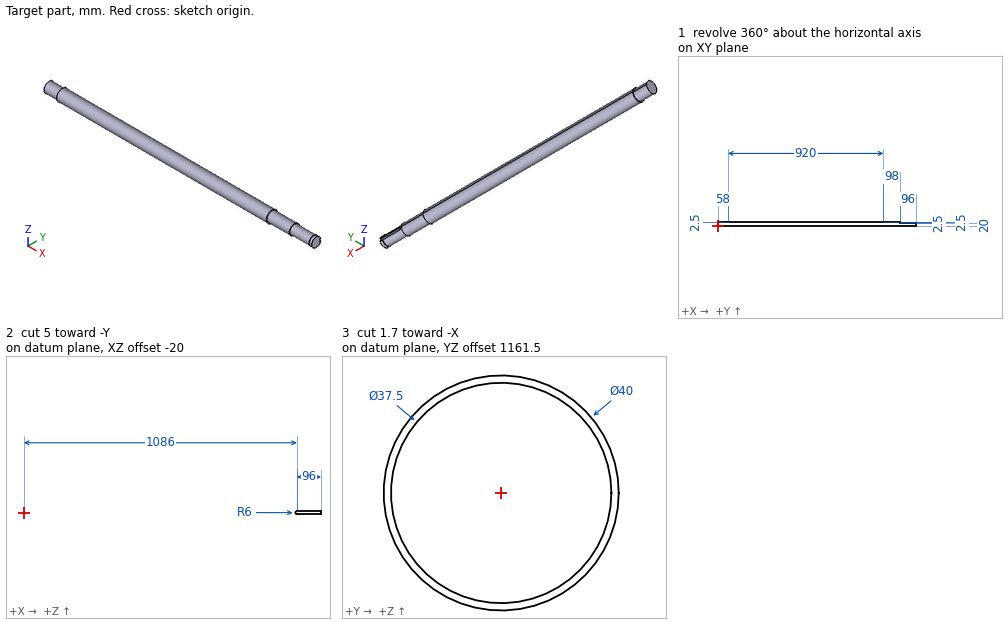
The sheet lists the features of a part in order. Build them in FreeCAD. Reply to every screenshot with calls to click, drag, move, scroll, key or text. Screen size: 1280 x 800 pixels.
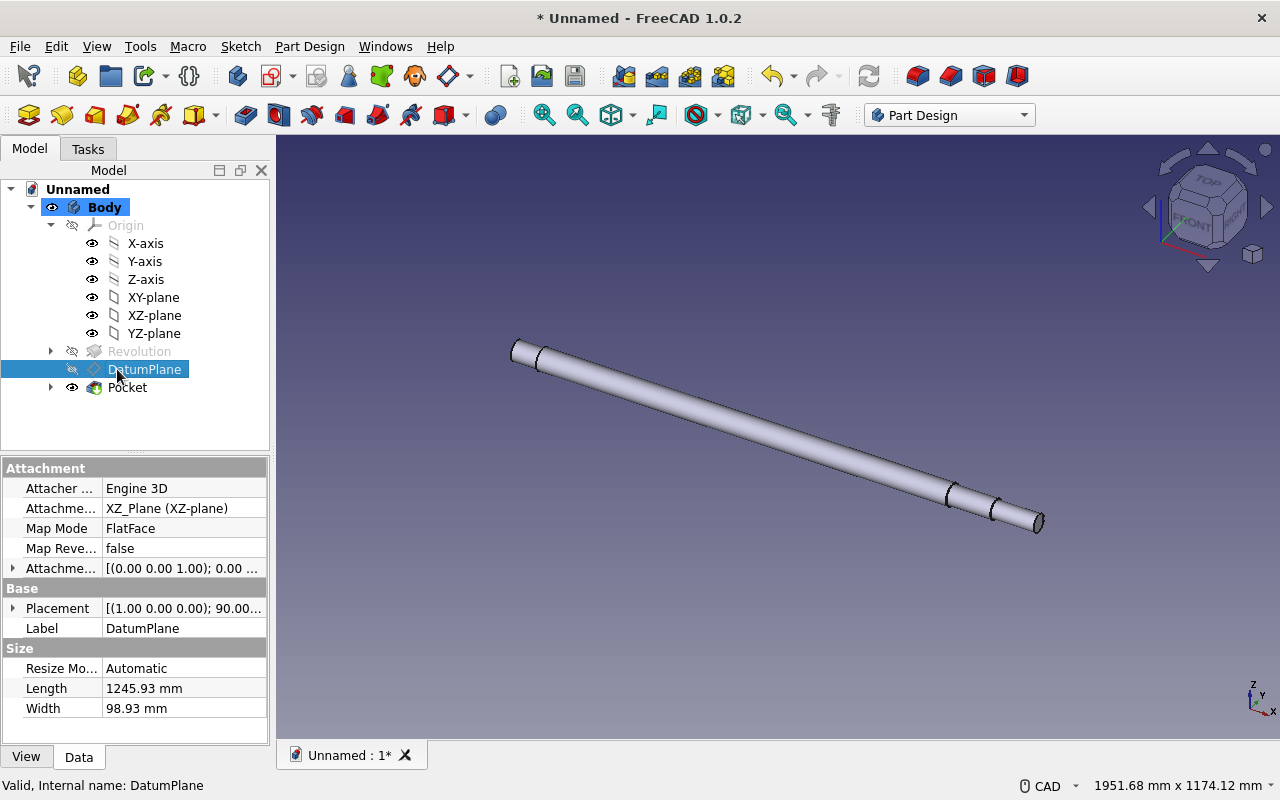
click(137, 333)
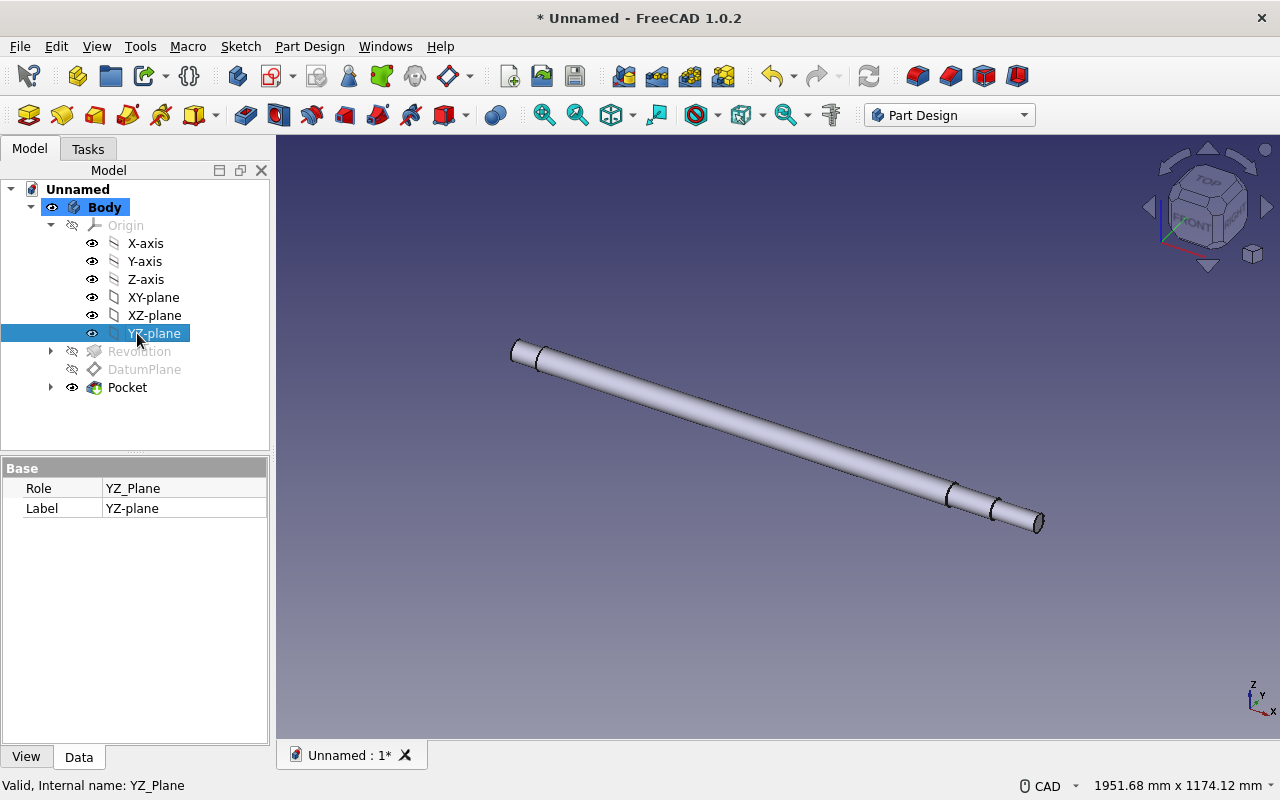
click(448, 76)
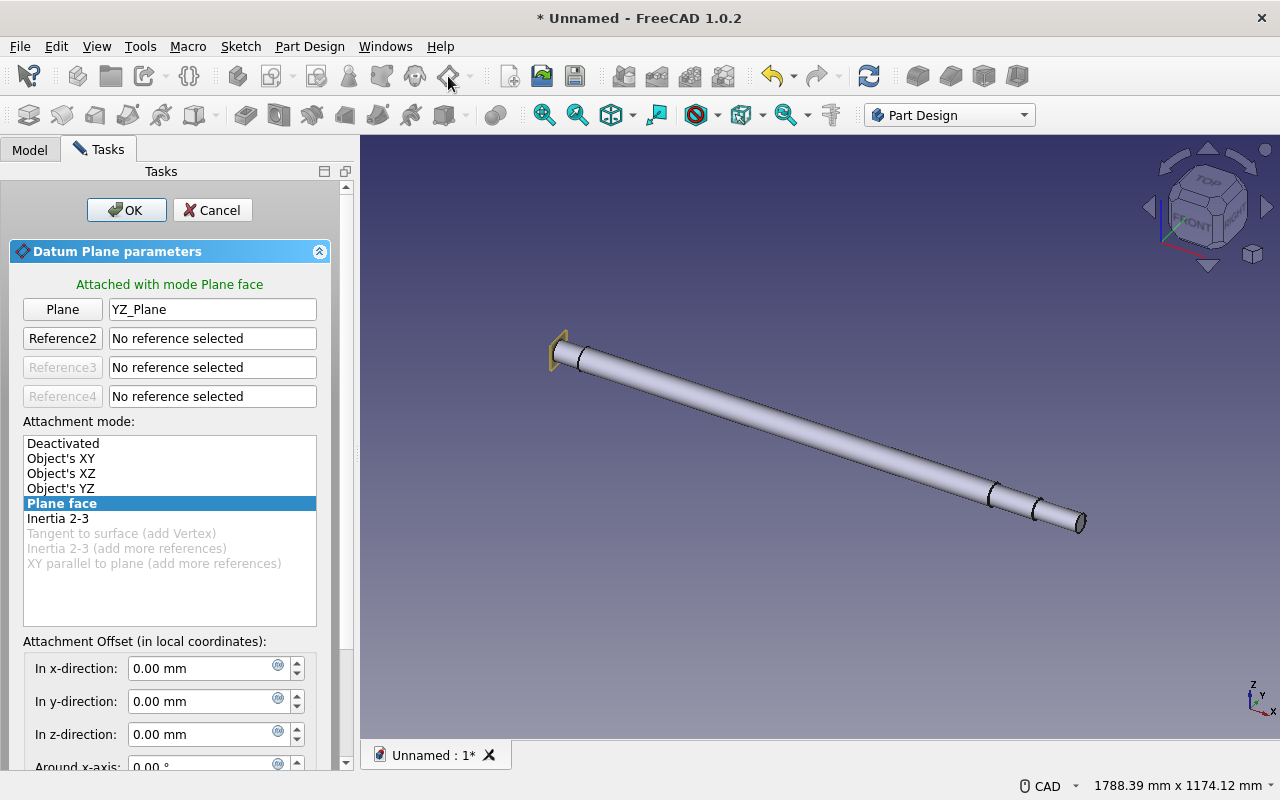
triple_click(210, 734)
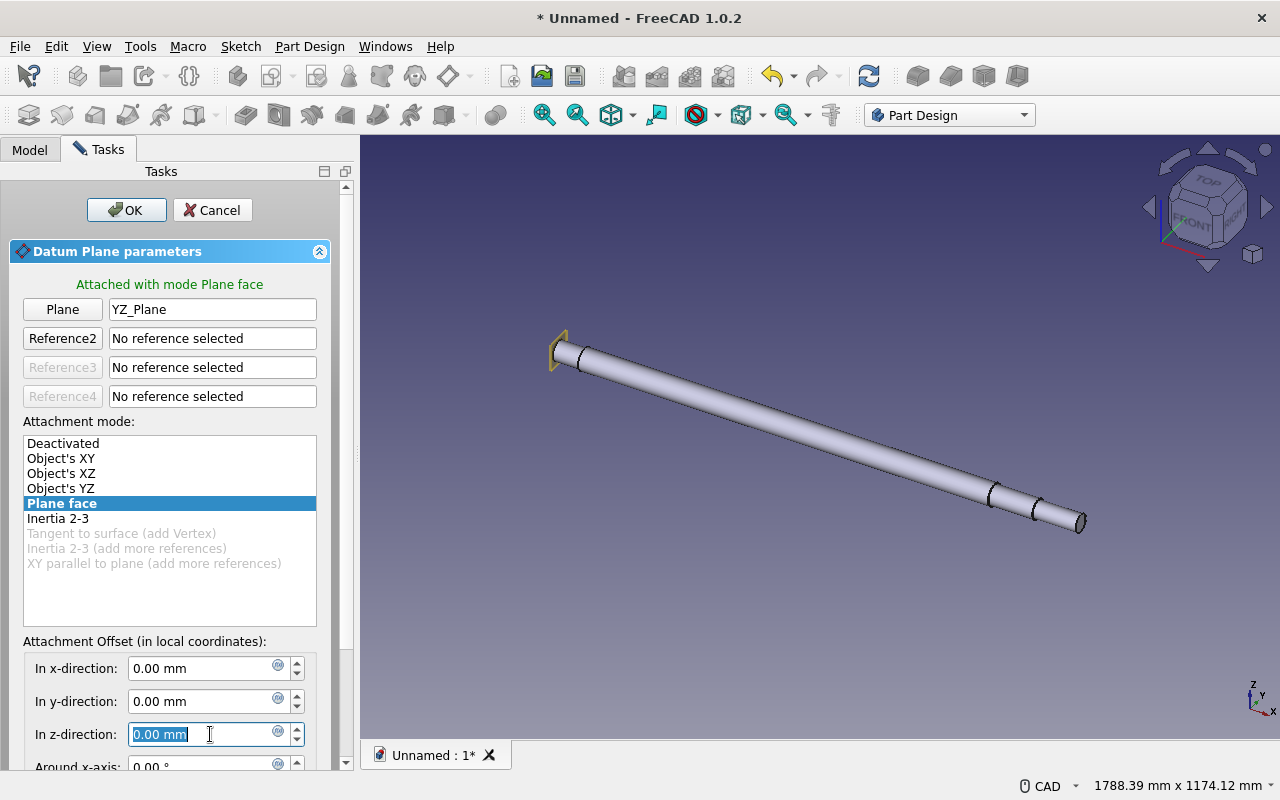
text(1161.5)
key(Tab)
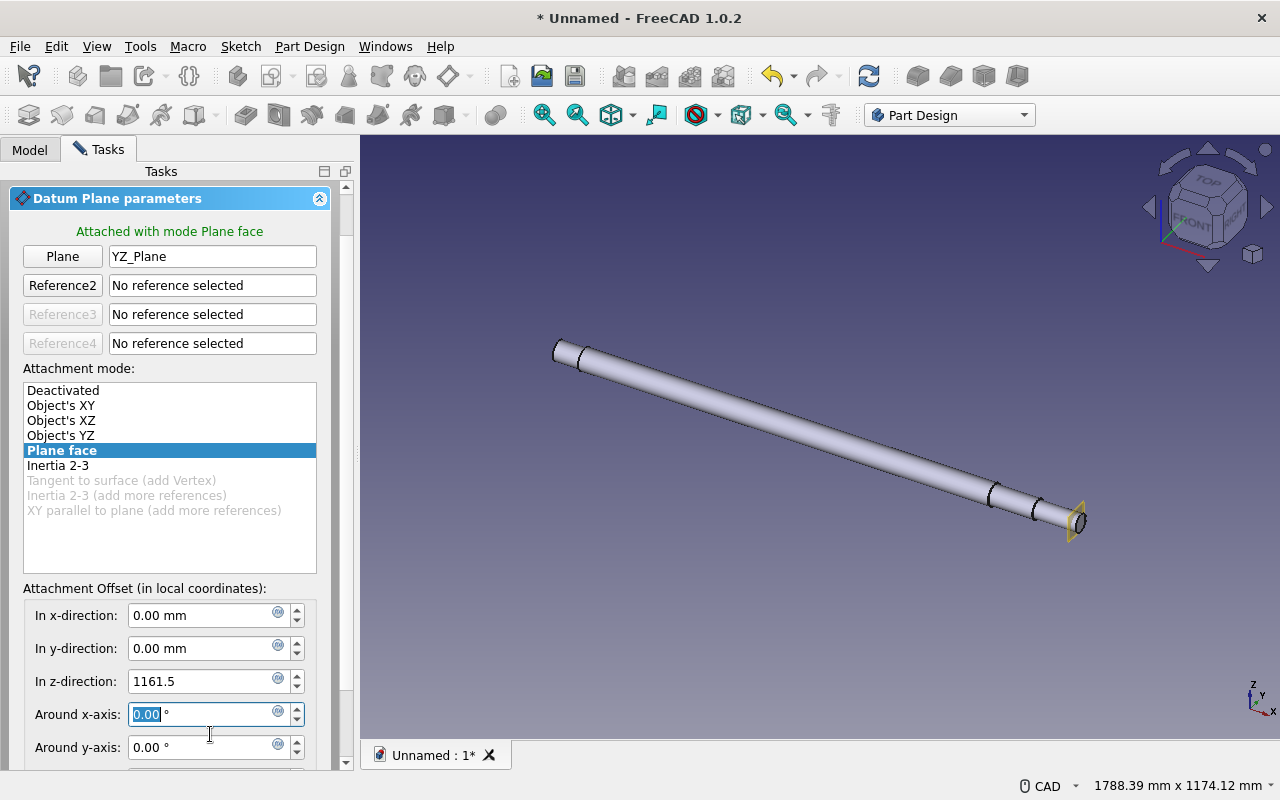
scroll(346, 476, up, 2)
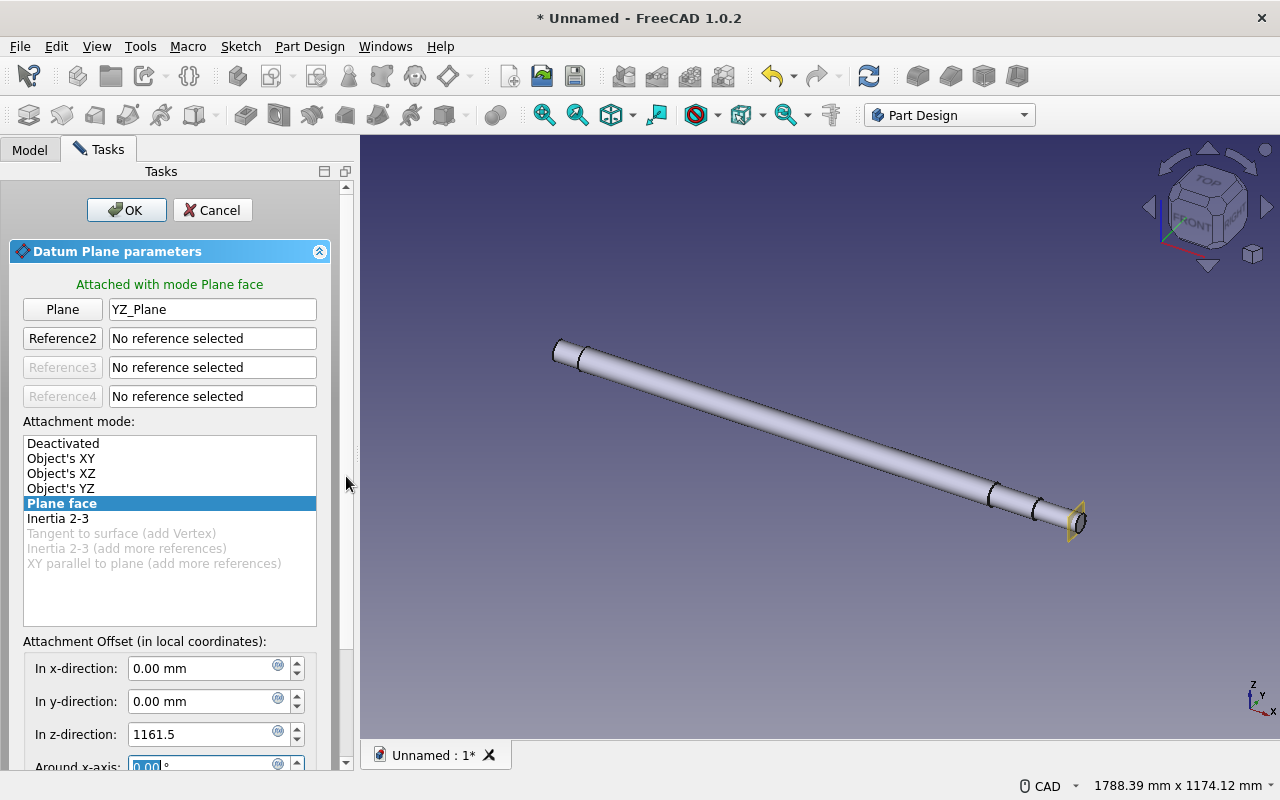
click(127, 210)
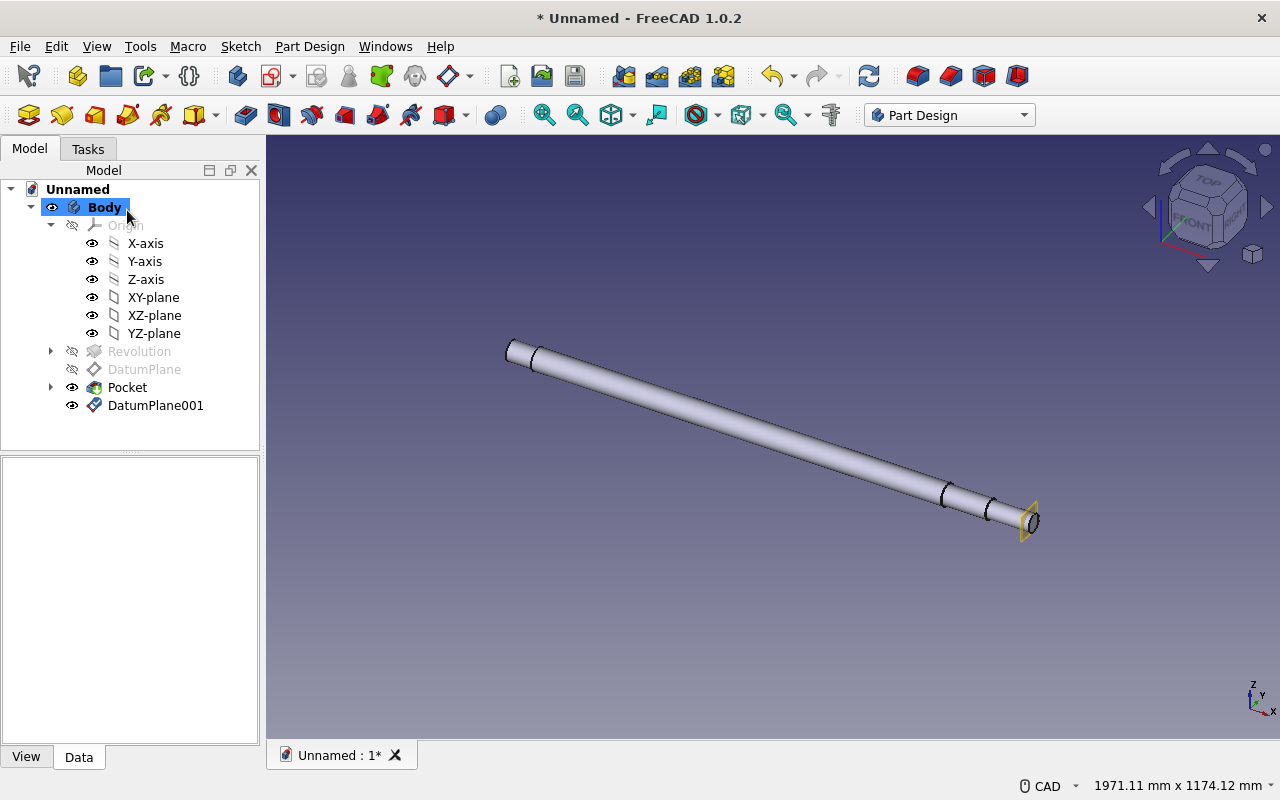
click(117, 405)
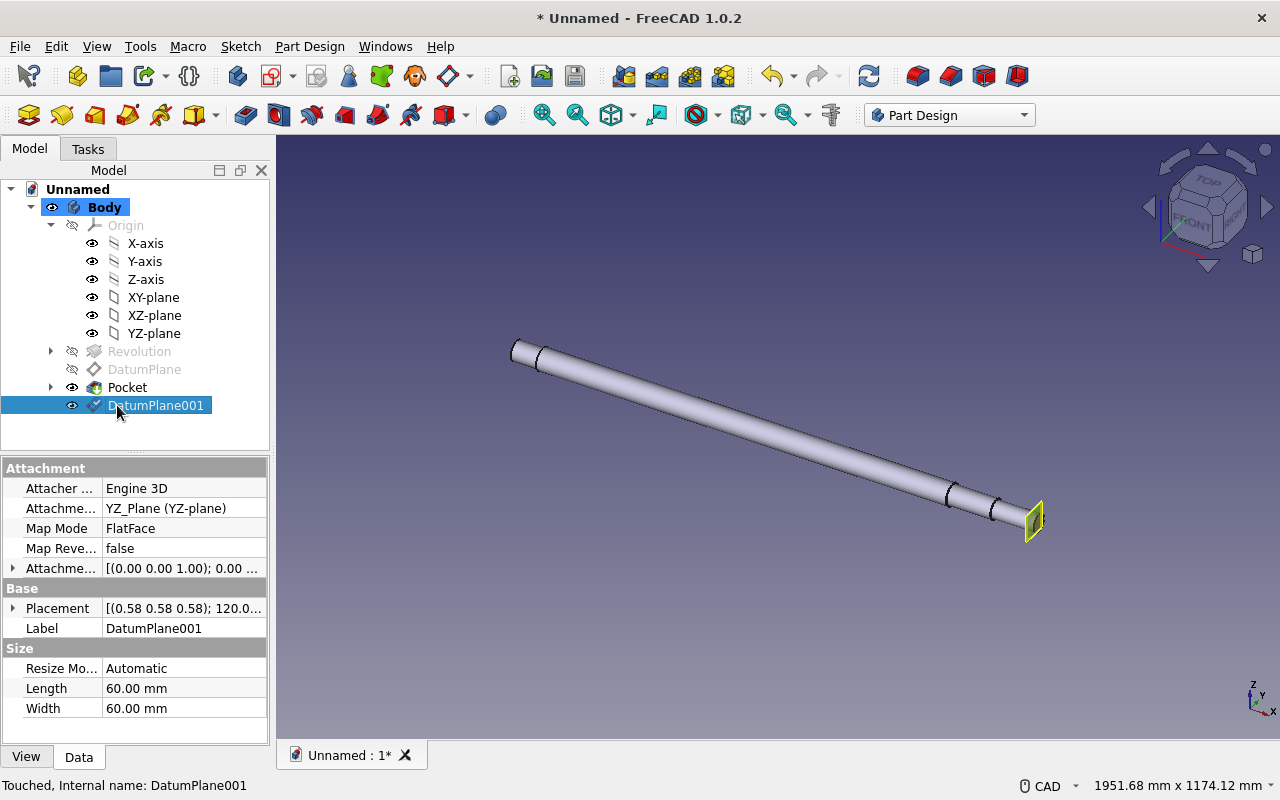
click(270, 76)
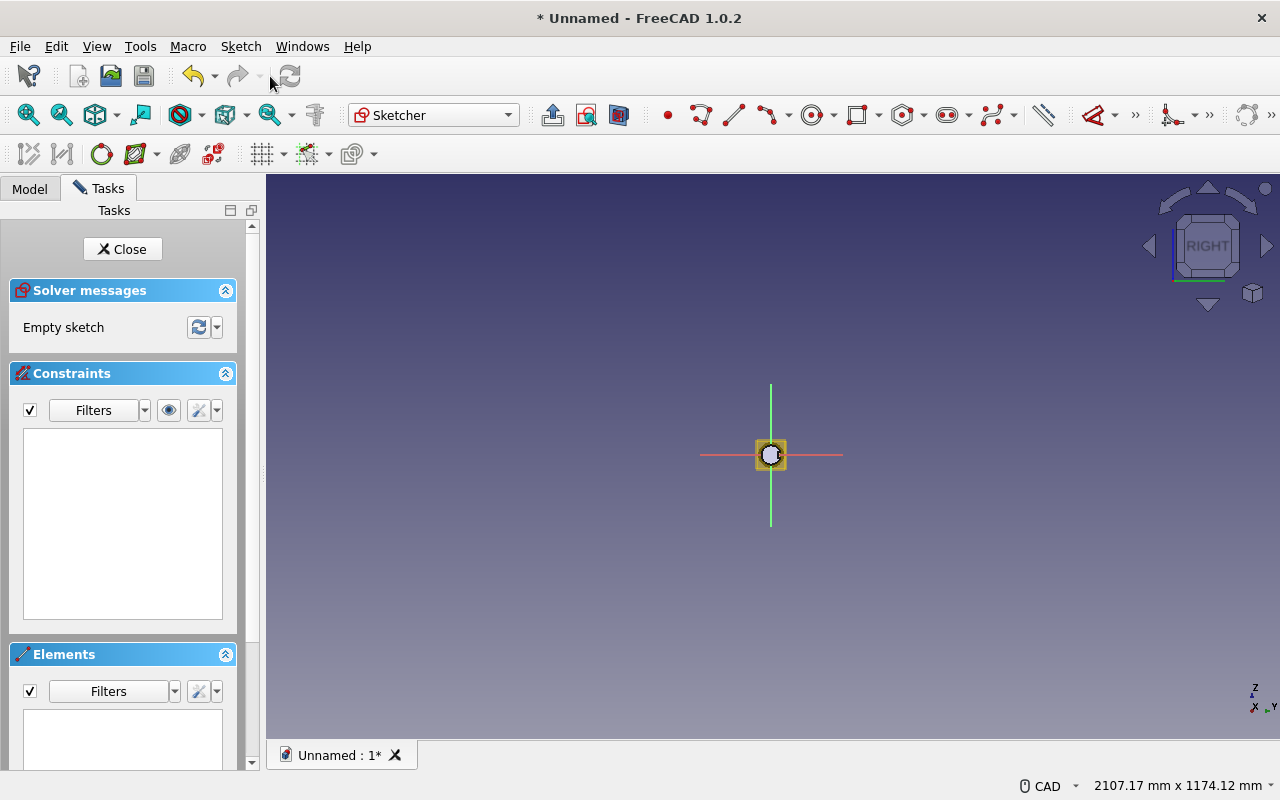
key(q)
key(s)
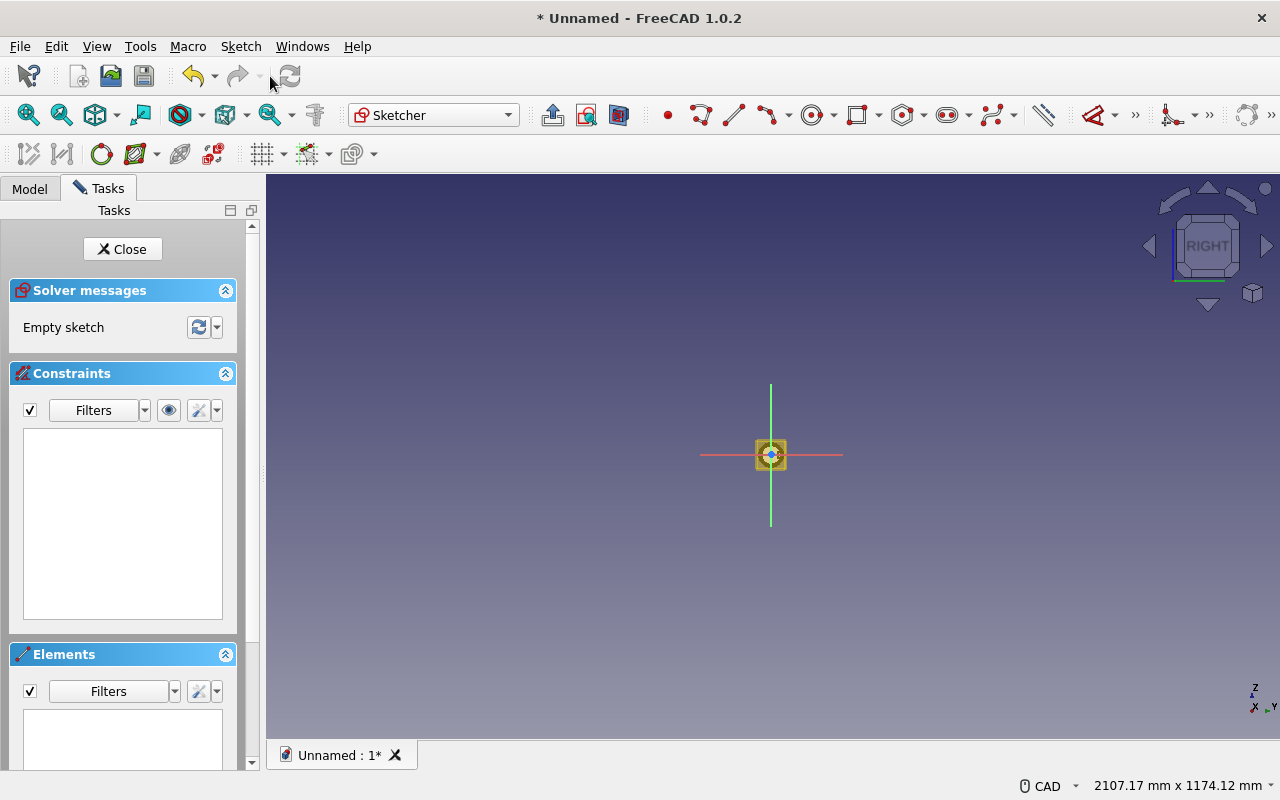
scroll(775, 455, up, 15)